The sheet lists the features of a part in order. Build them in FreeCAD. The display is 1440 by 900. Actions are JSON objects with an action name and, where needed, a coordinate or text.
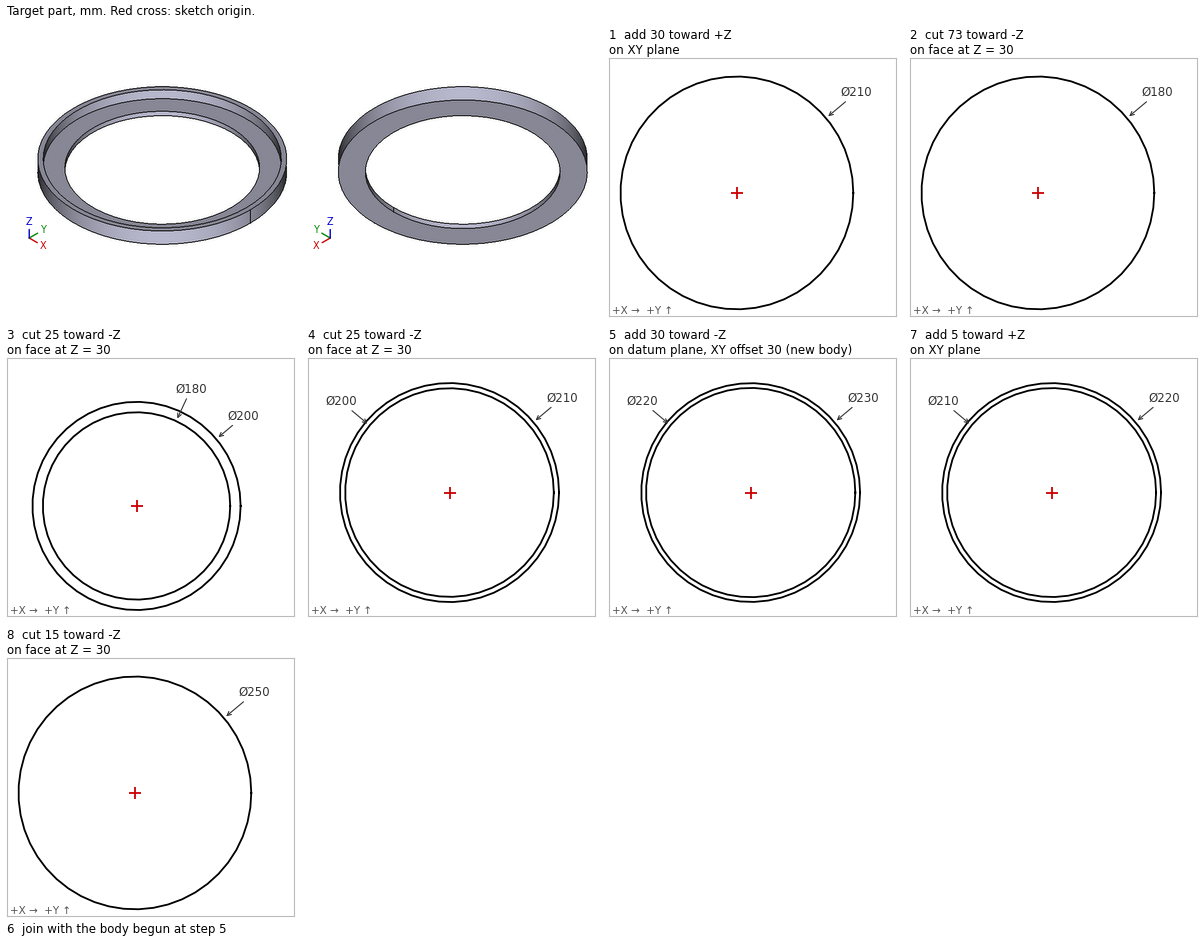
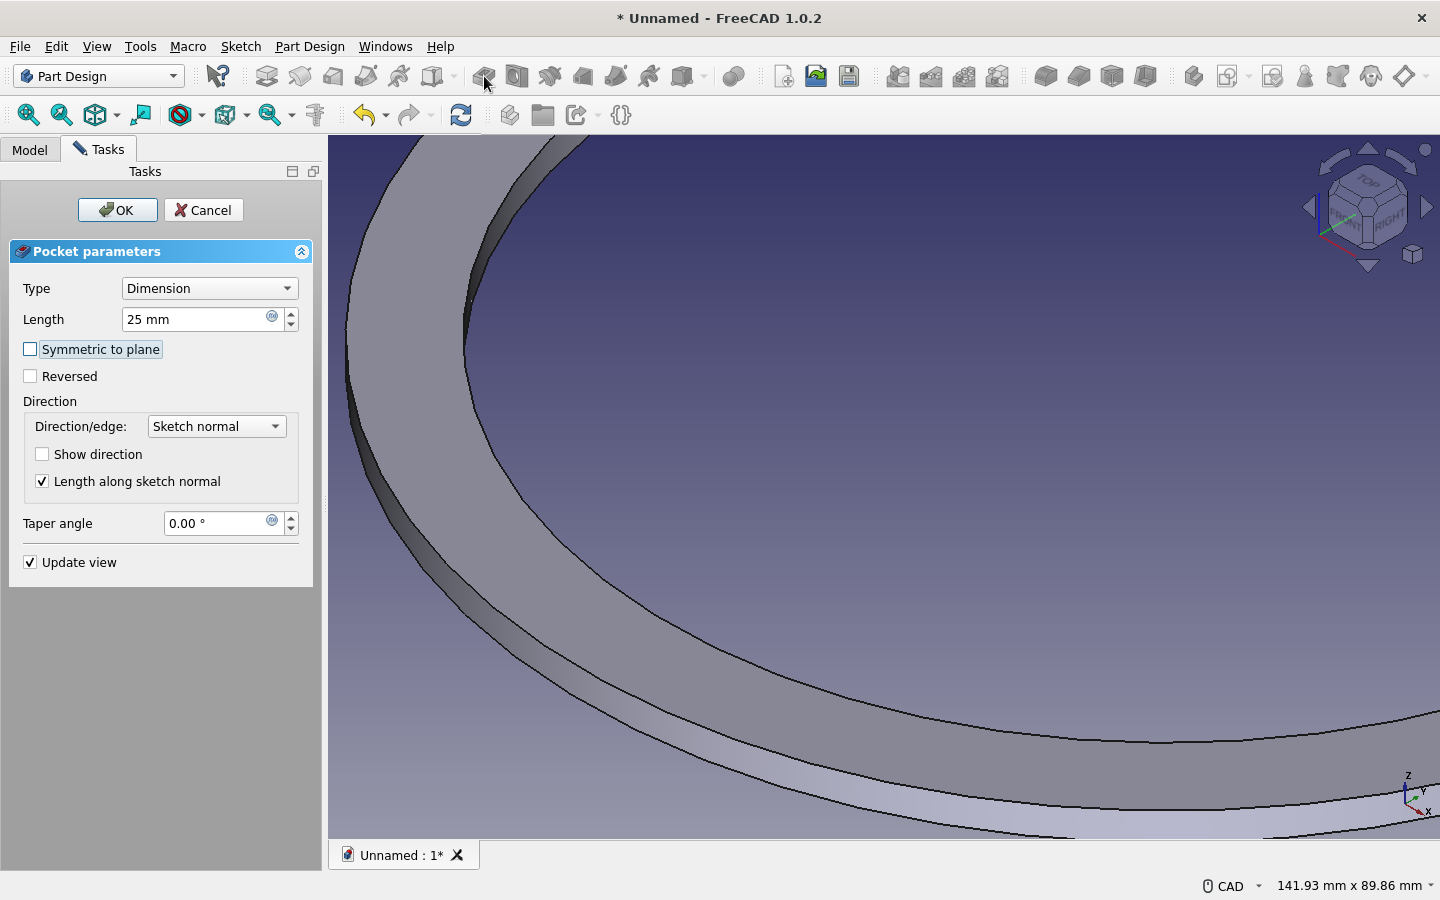
{"action": "left_click", "coordinate": [118, 210]}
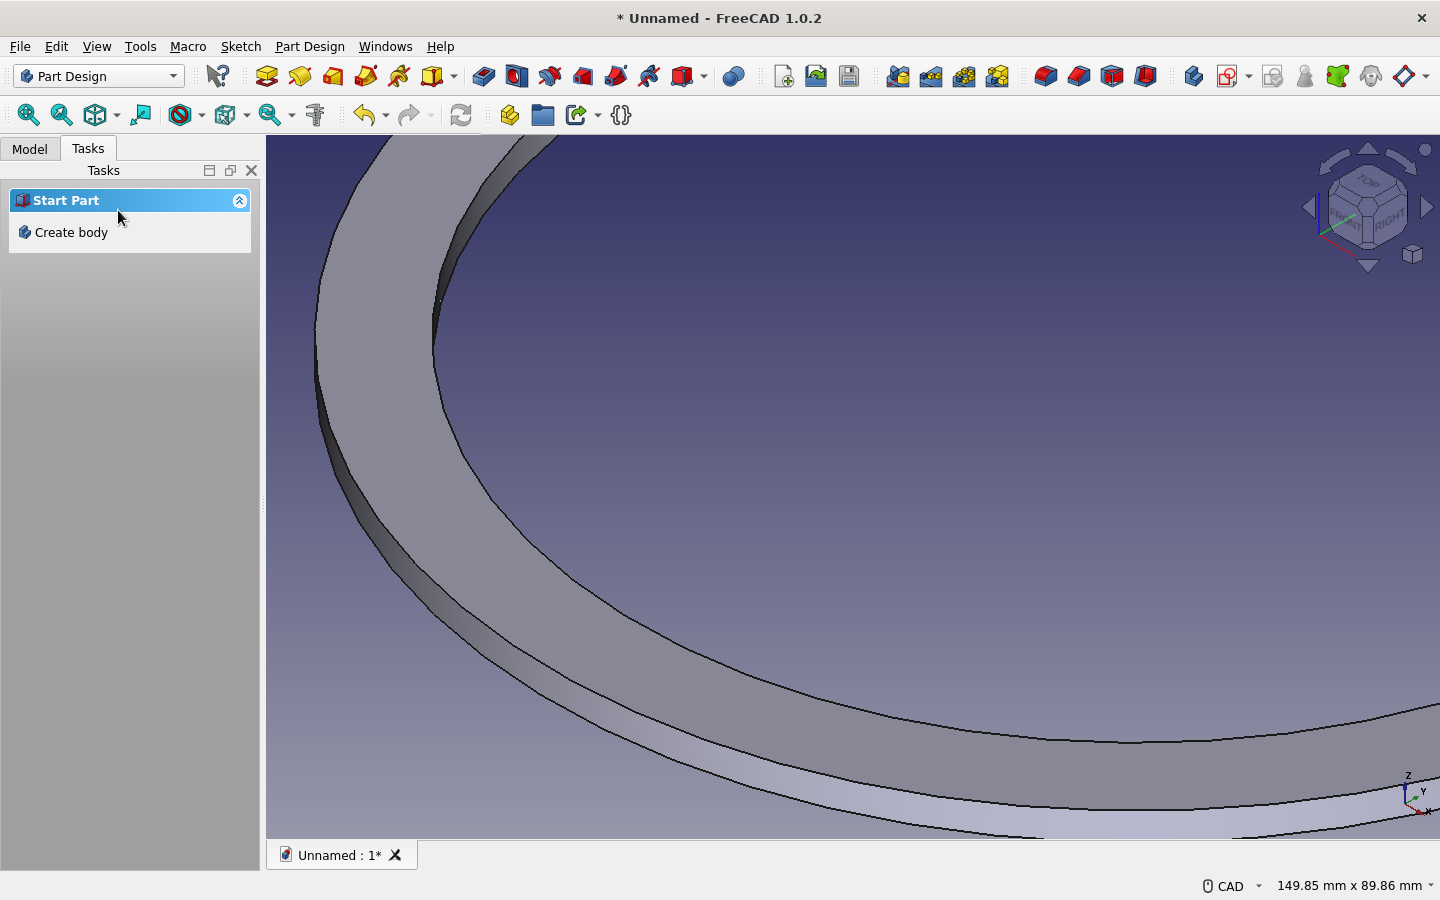
{"action": "left_click", "coordinate": [29, 116]}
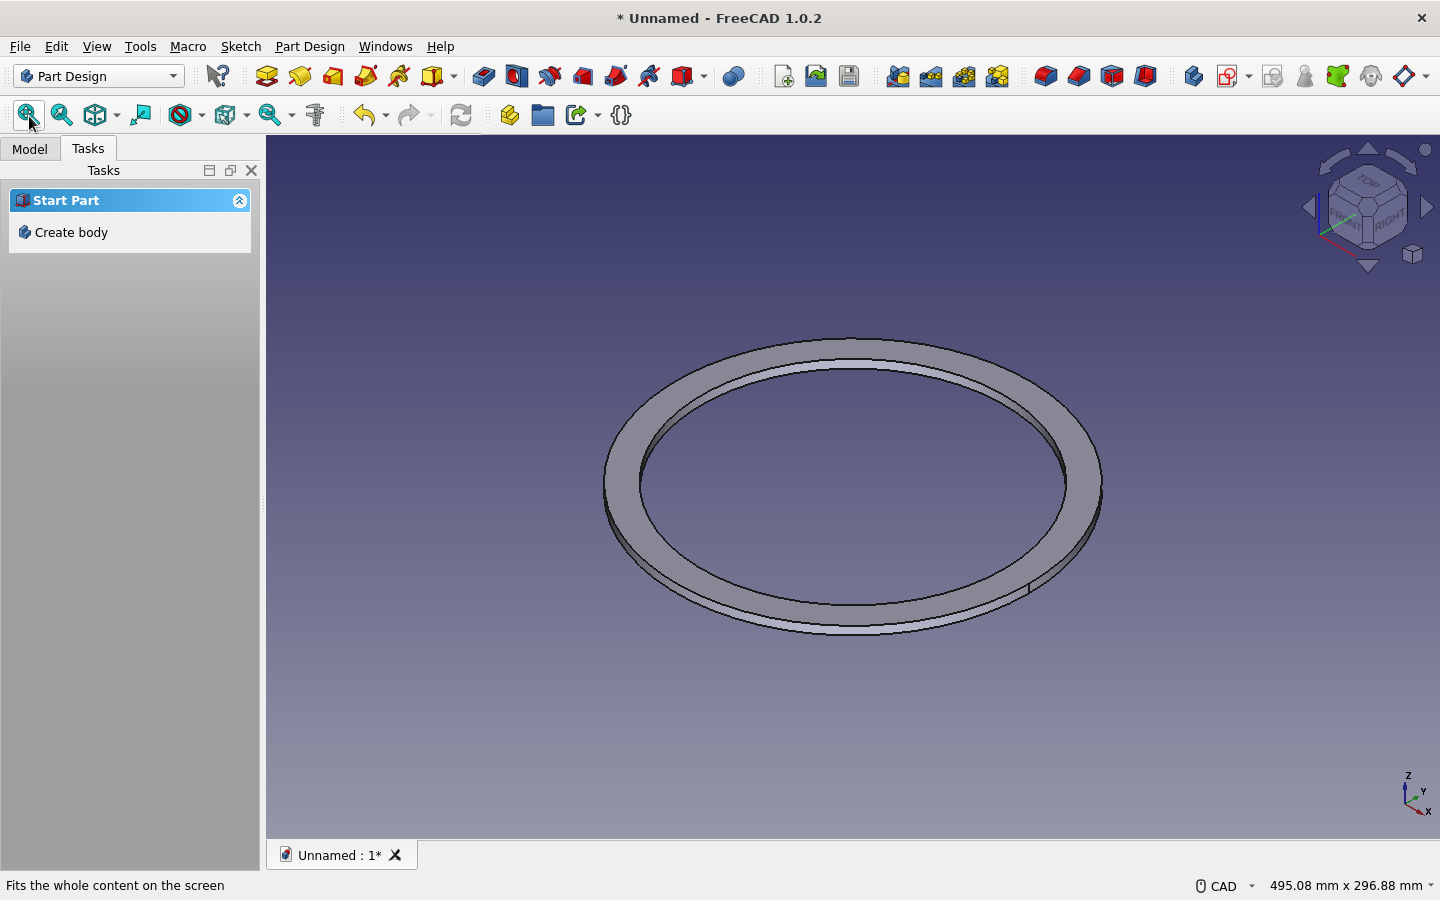
{"action": "left_click", "coordinate": [1194, 76]}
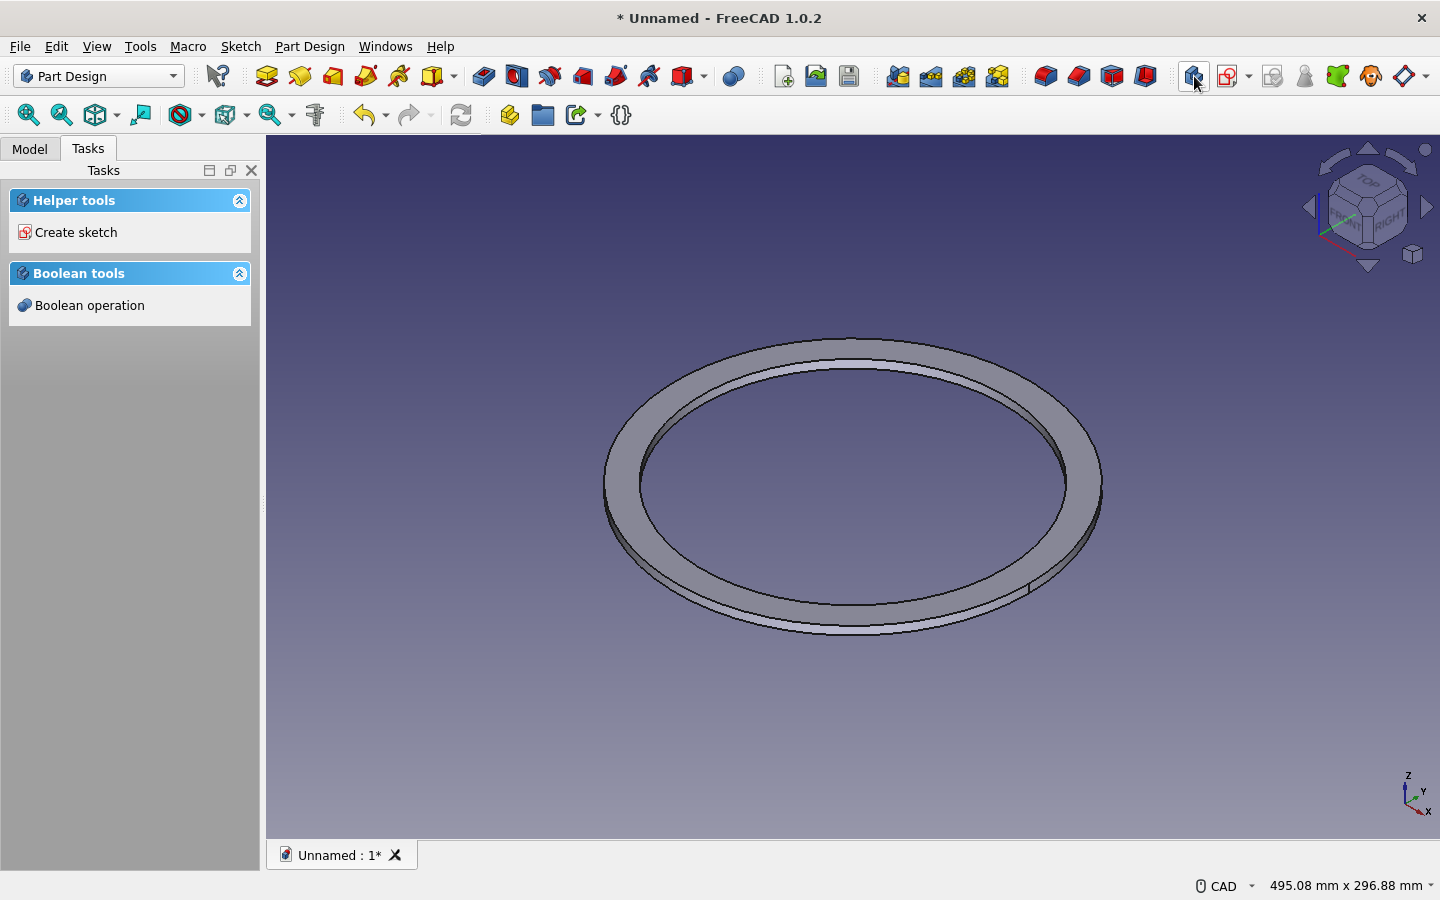
{"action": "left_click", "coordinate": [30, 148]}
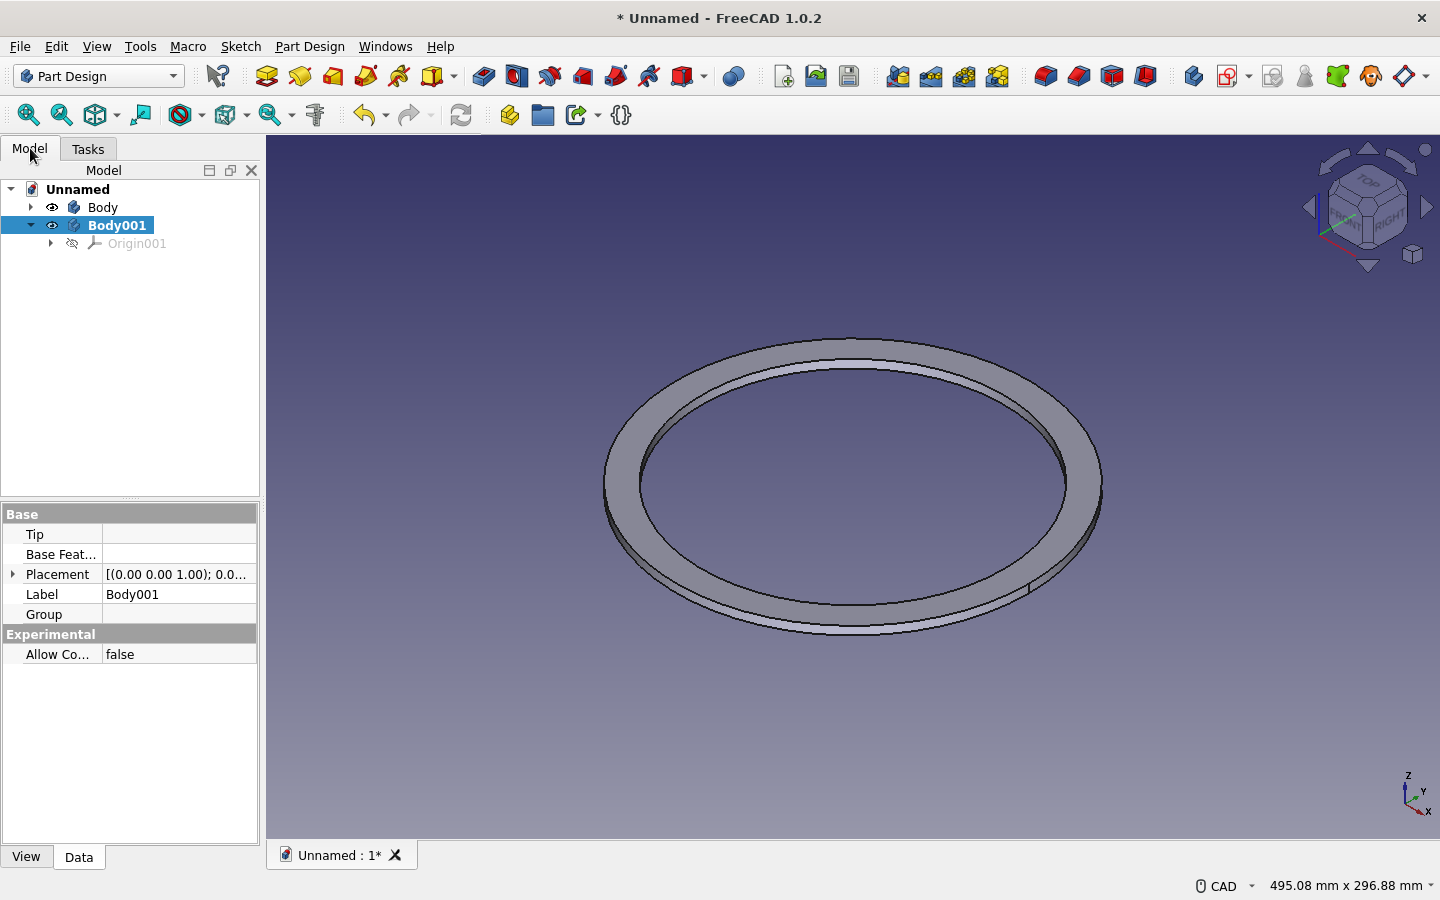
{"action": "left_click", "coordinate": [51, 243]}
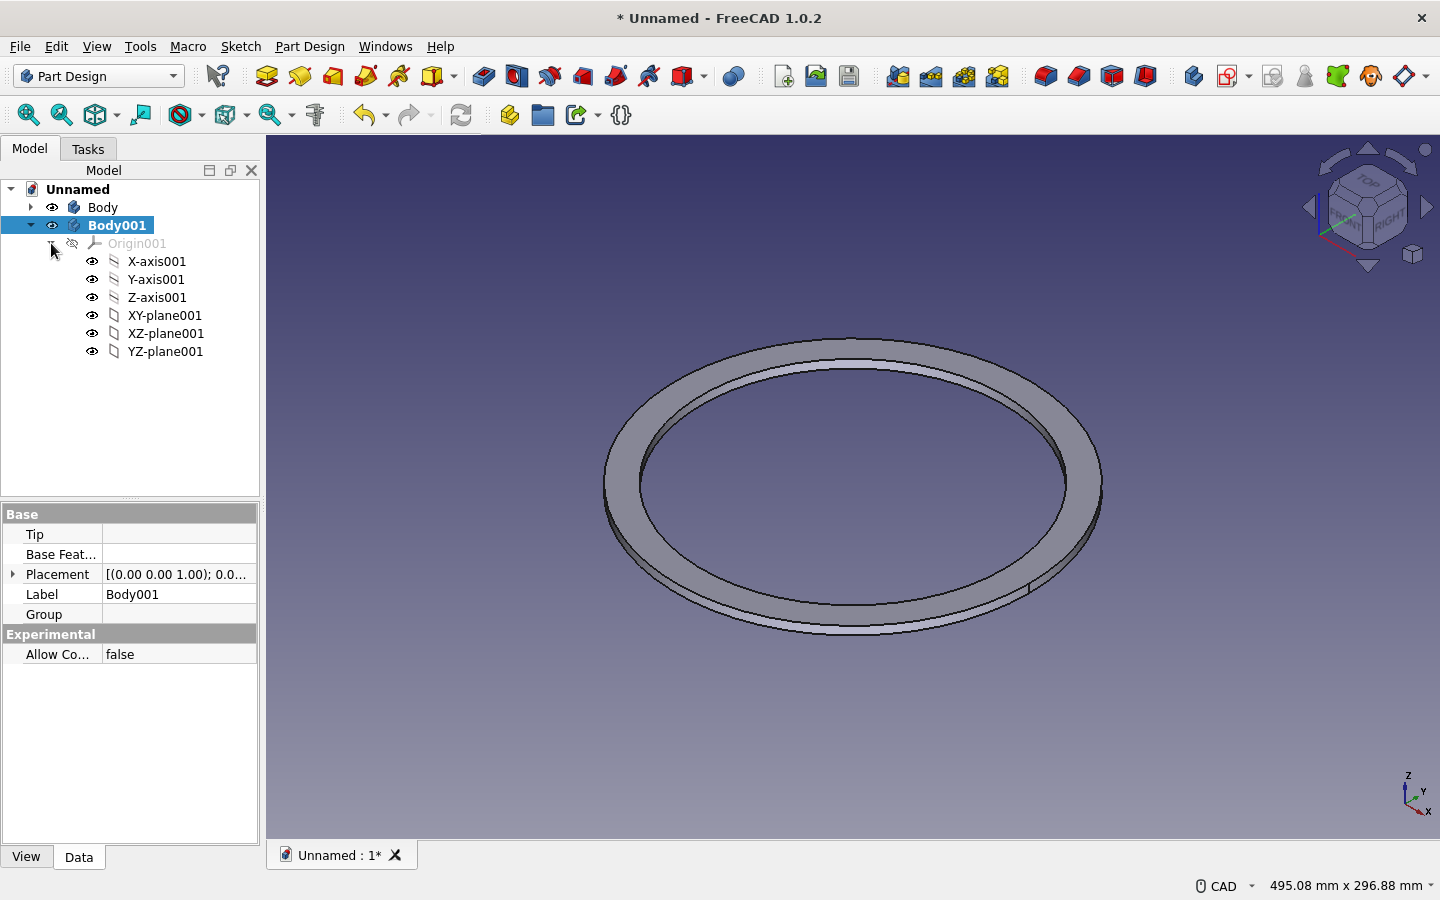
{"action": "left_click", "coordinate": [137, 315]}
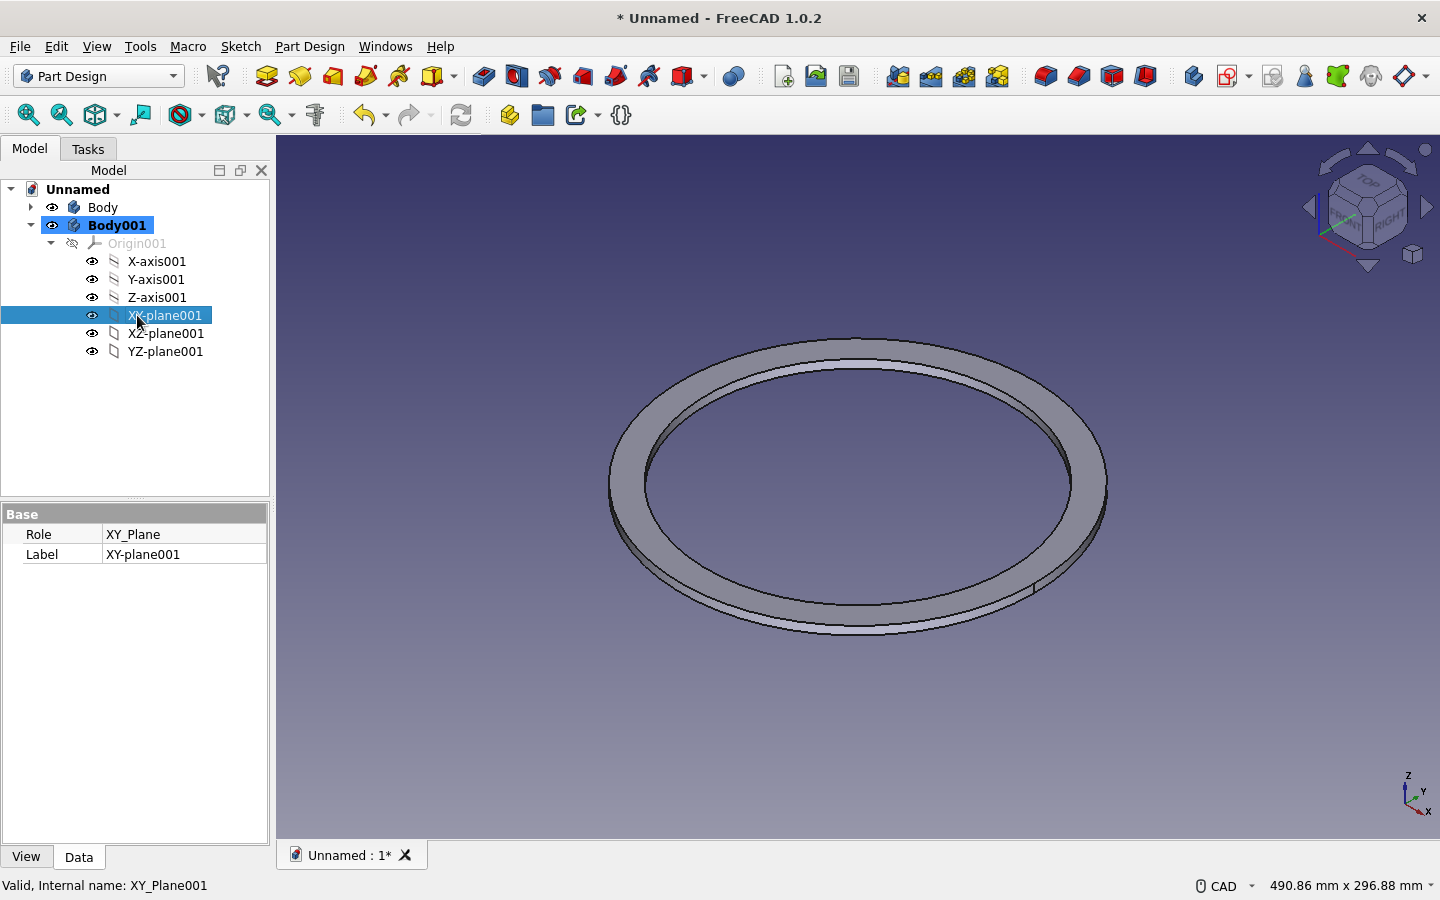
{"action": "left_click", "coordinate": [1404, 76]}